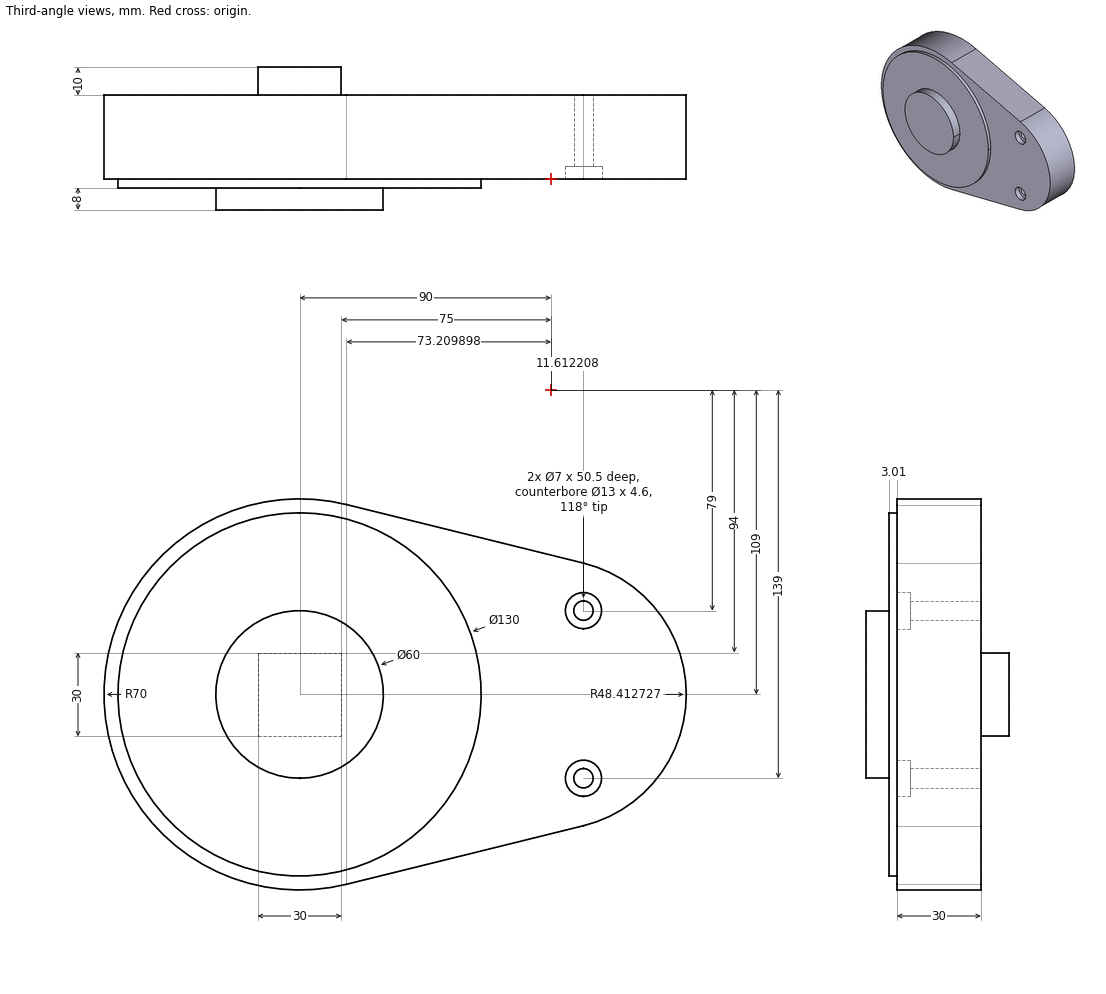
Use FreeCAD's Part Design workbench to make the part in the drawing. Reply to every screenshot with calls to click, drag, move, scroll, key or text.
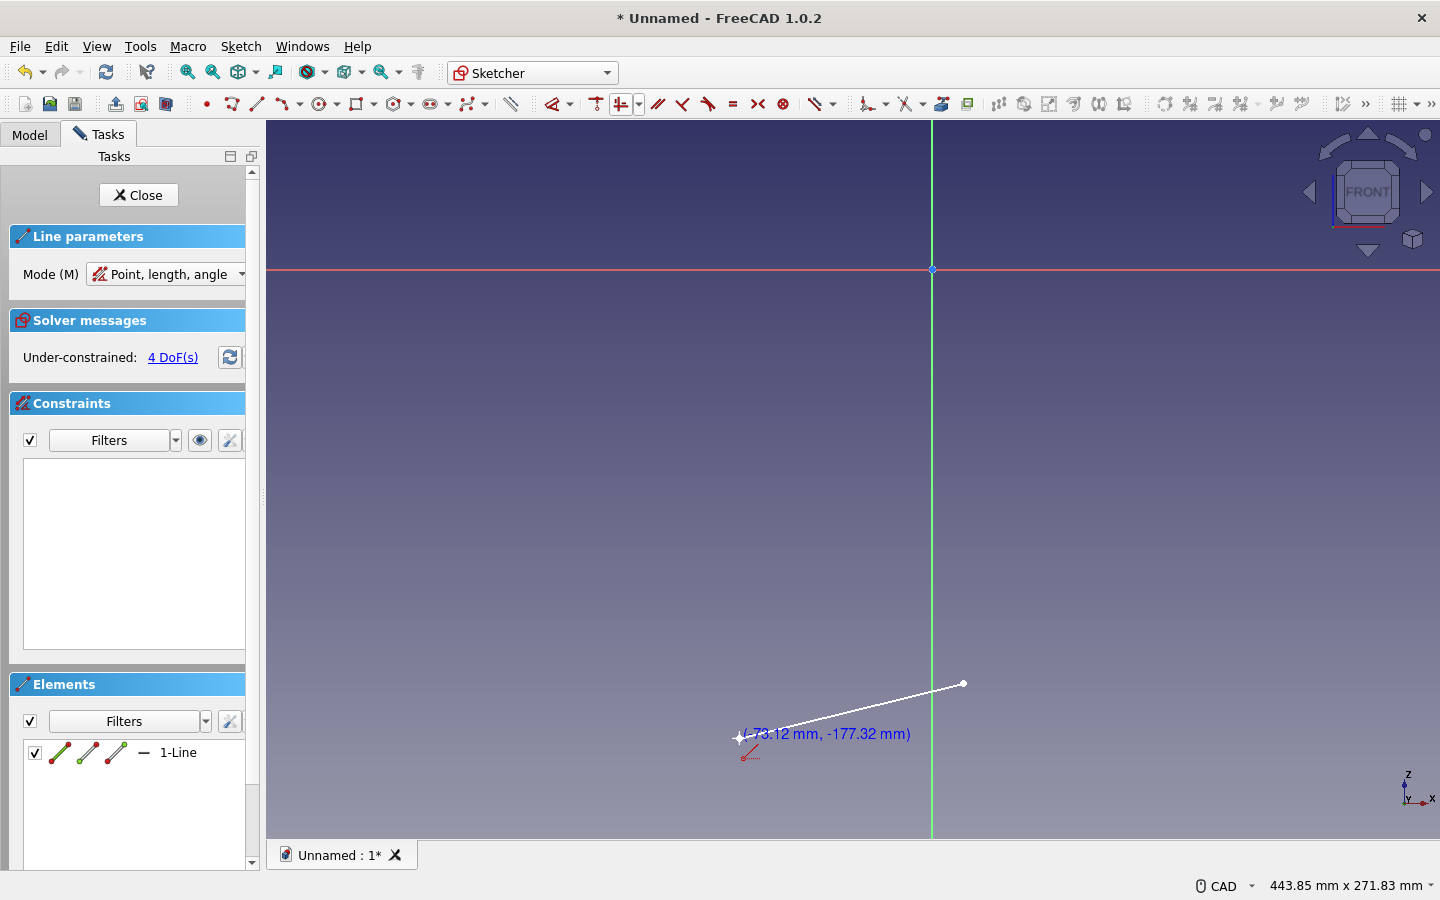
click(739, 379)
click(963, 434)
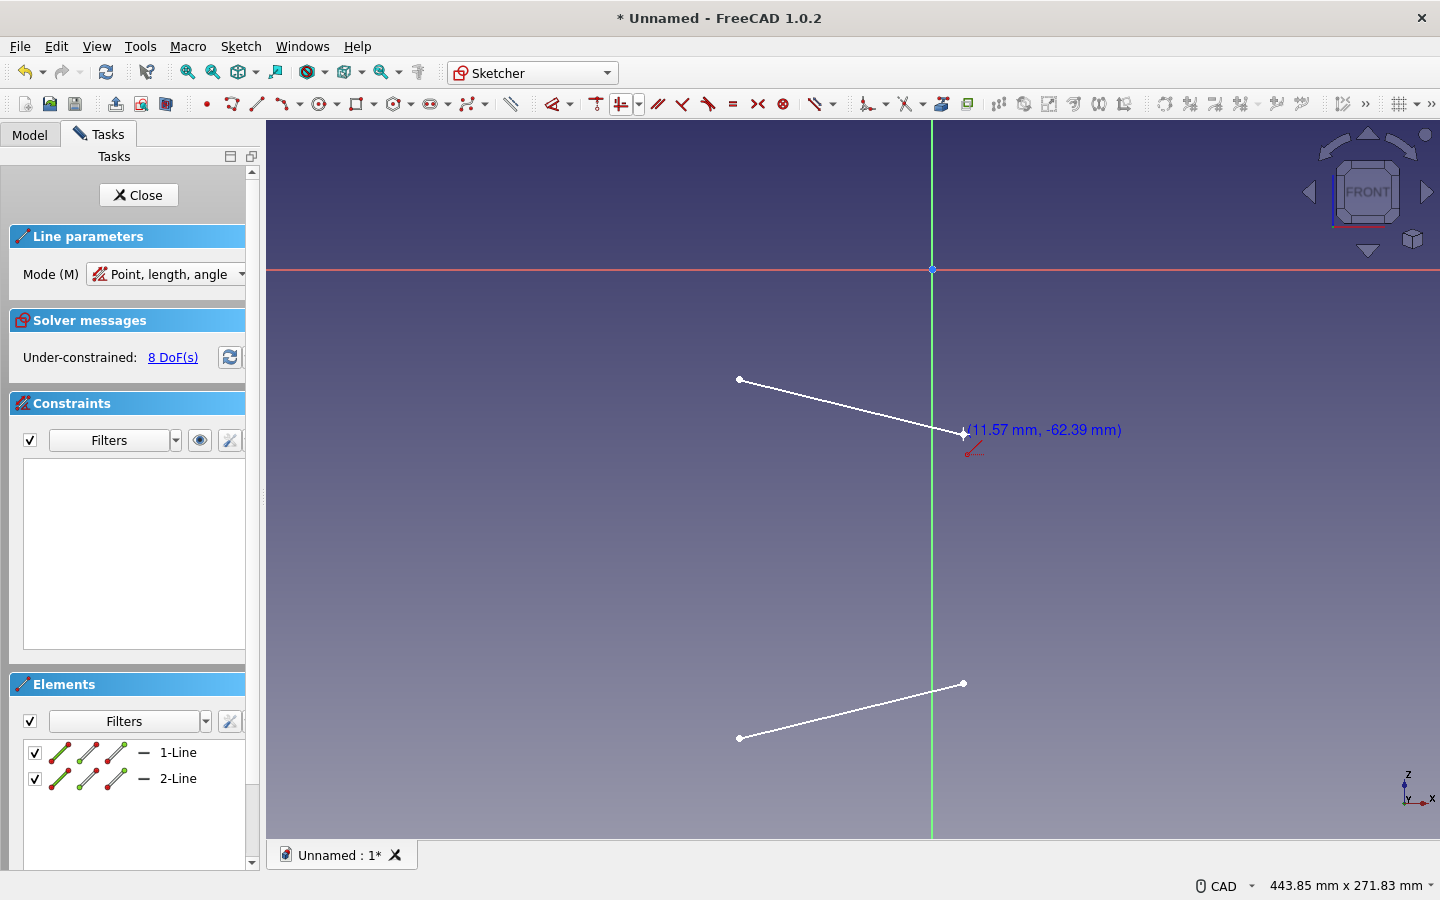
key(g)
key(3)
key(a)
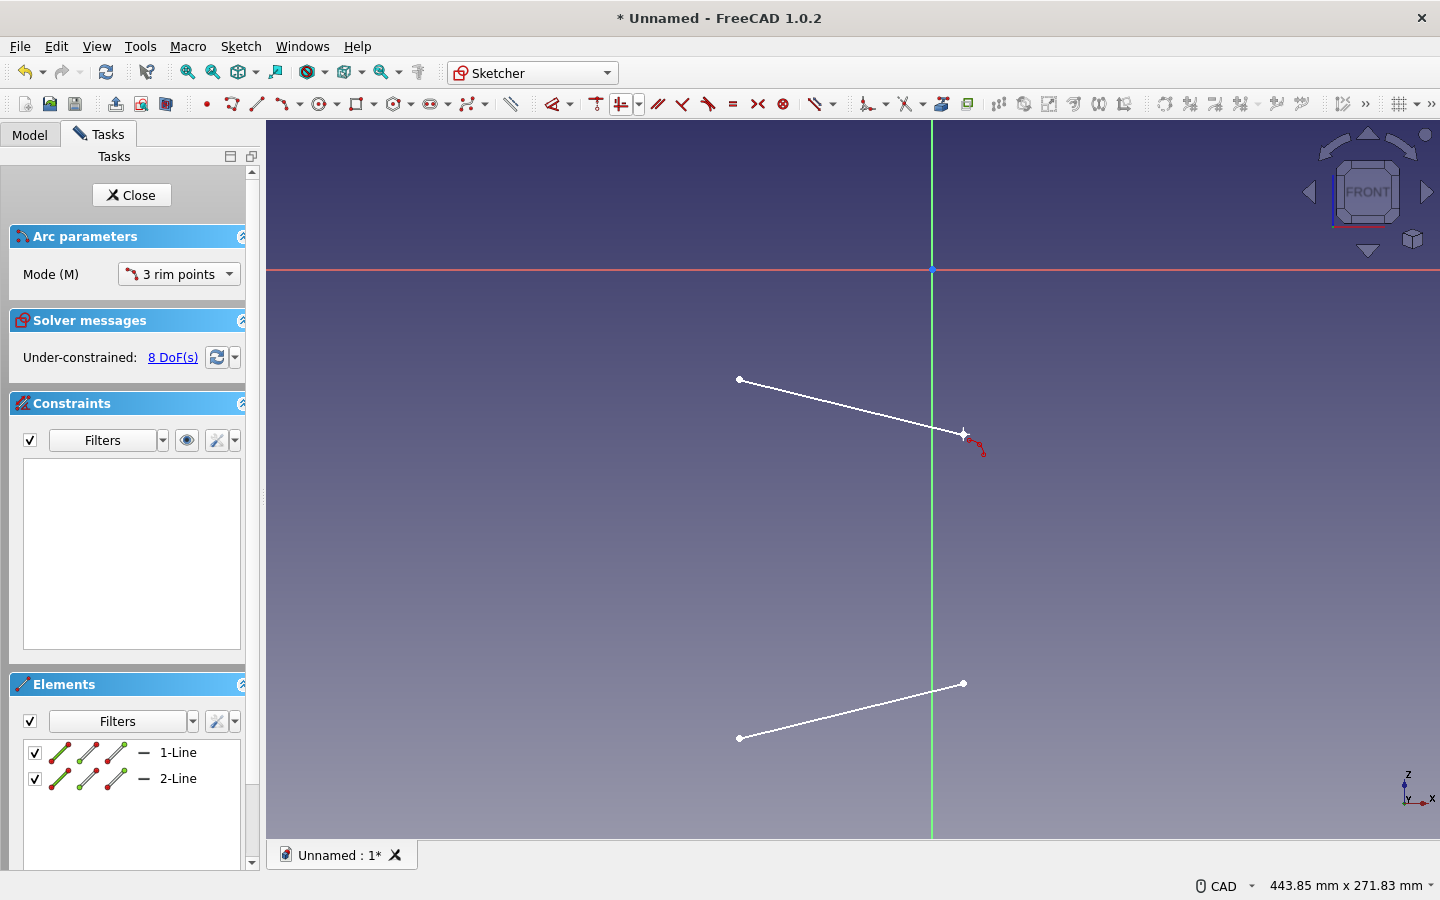
click(739, 739)
click(739, 380)
click(509, 558)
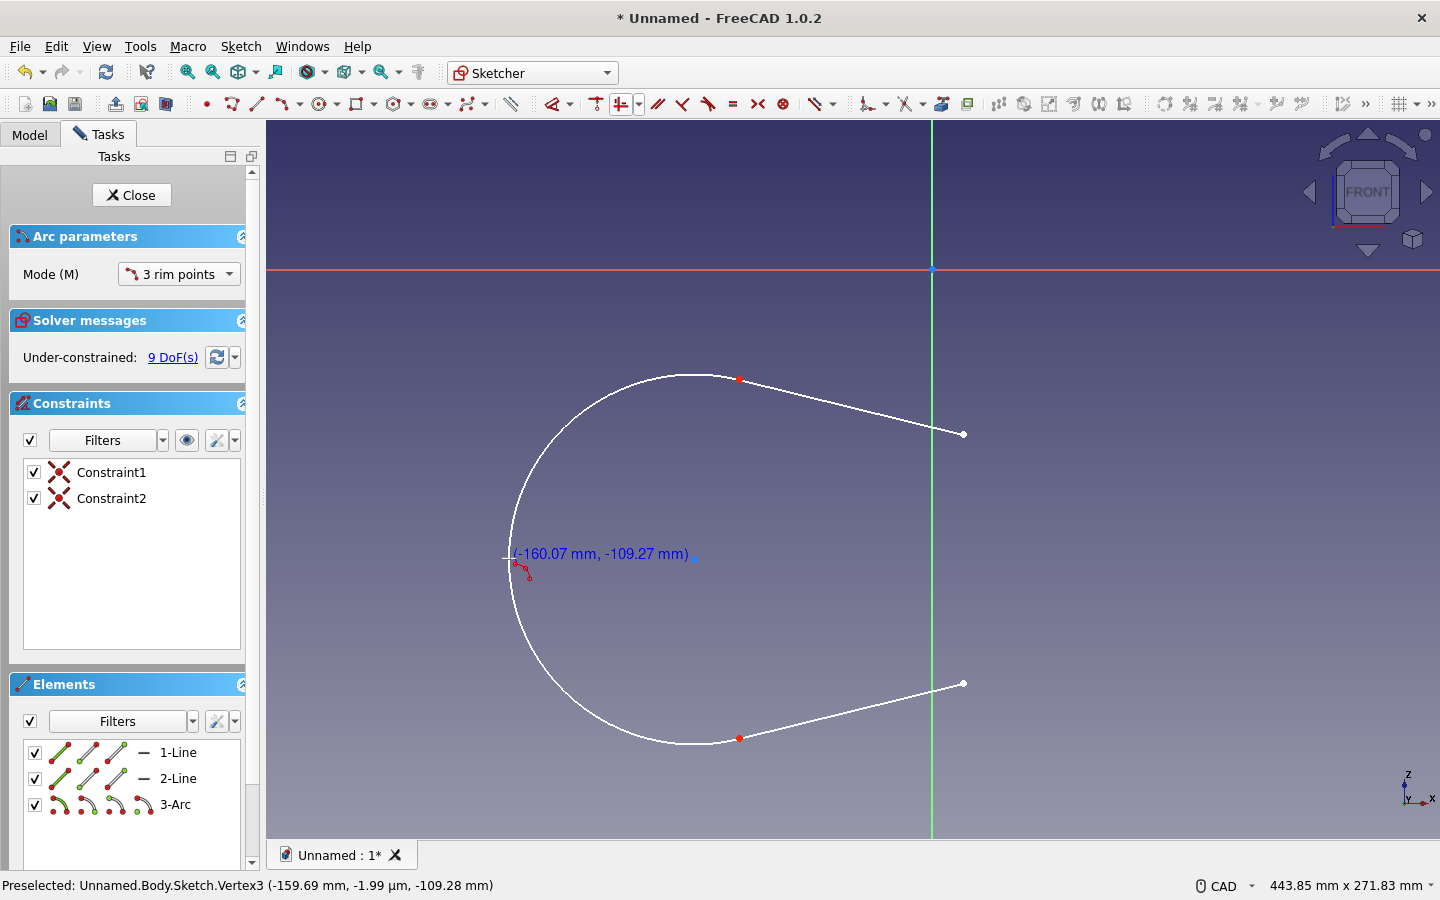
click(963, 435)
click(963, 684)
click(1060, 558)
key(Escape)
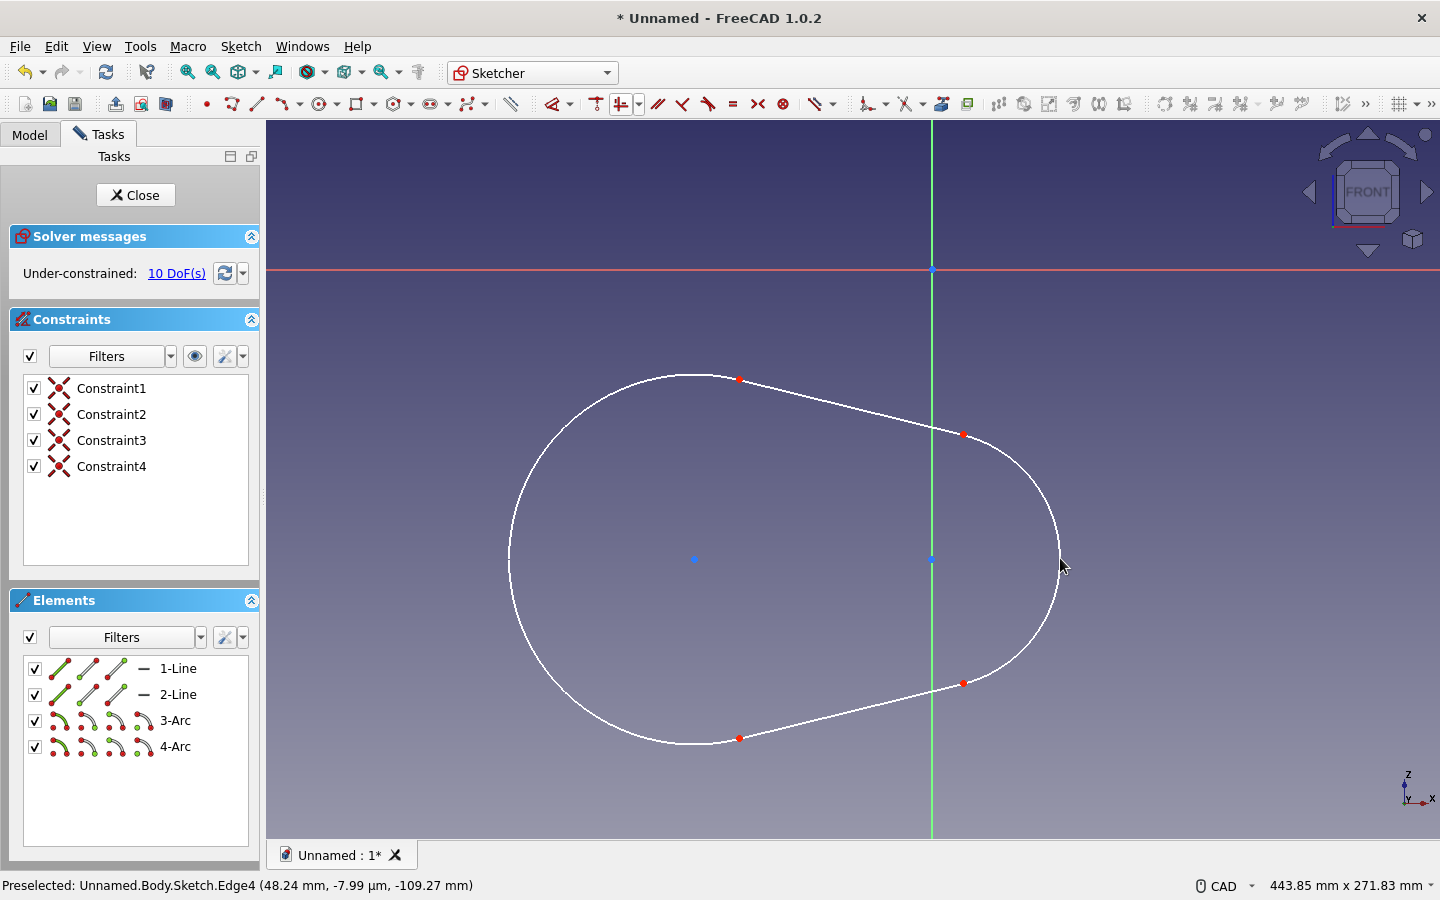
click(896, 701)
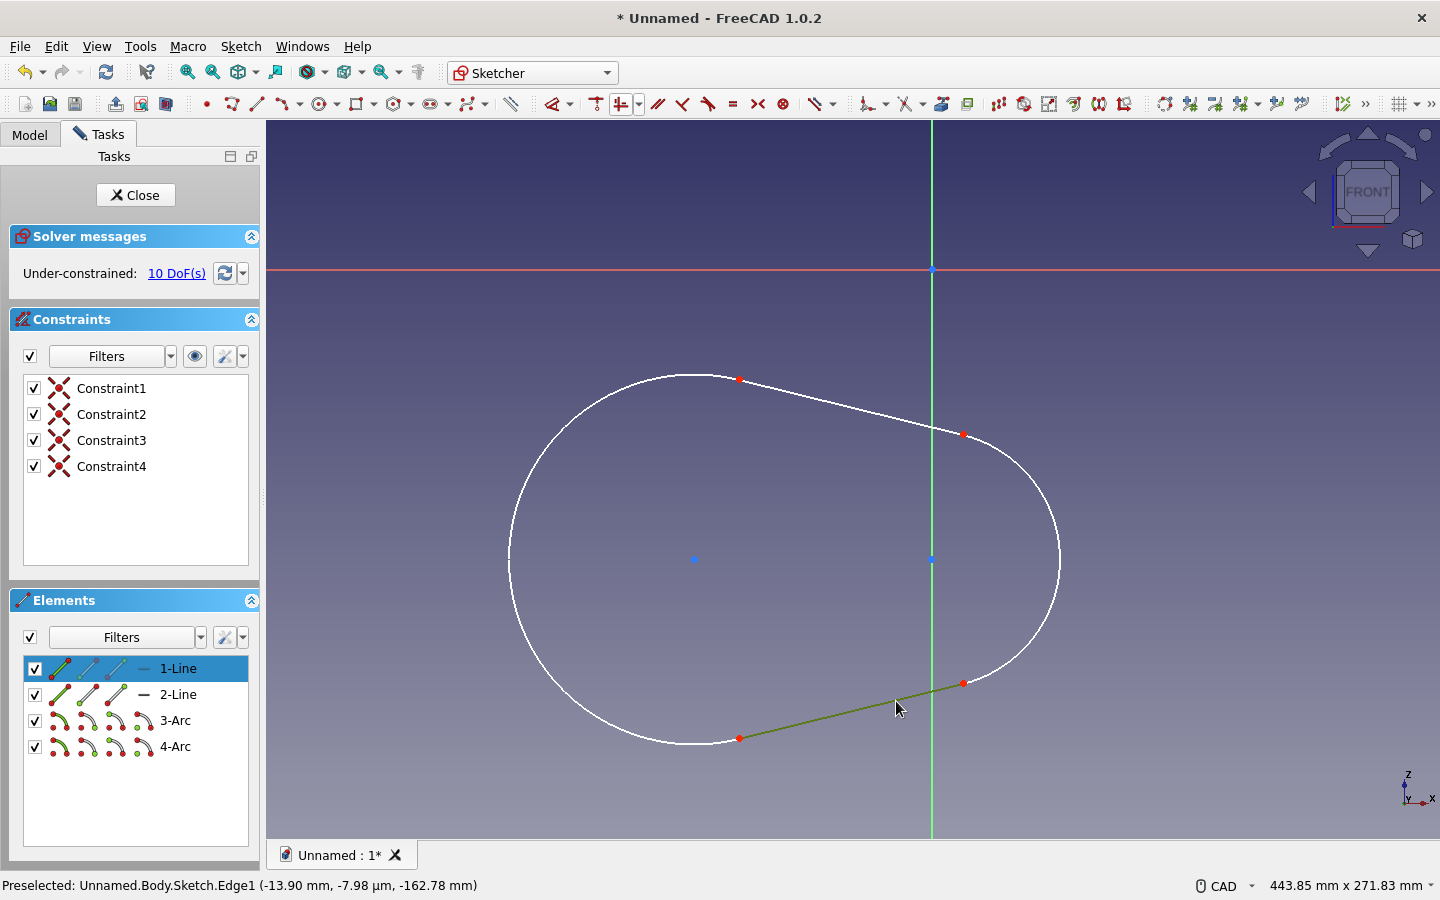
click(1042, 624)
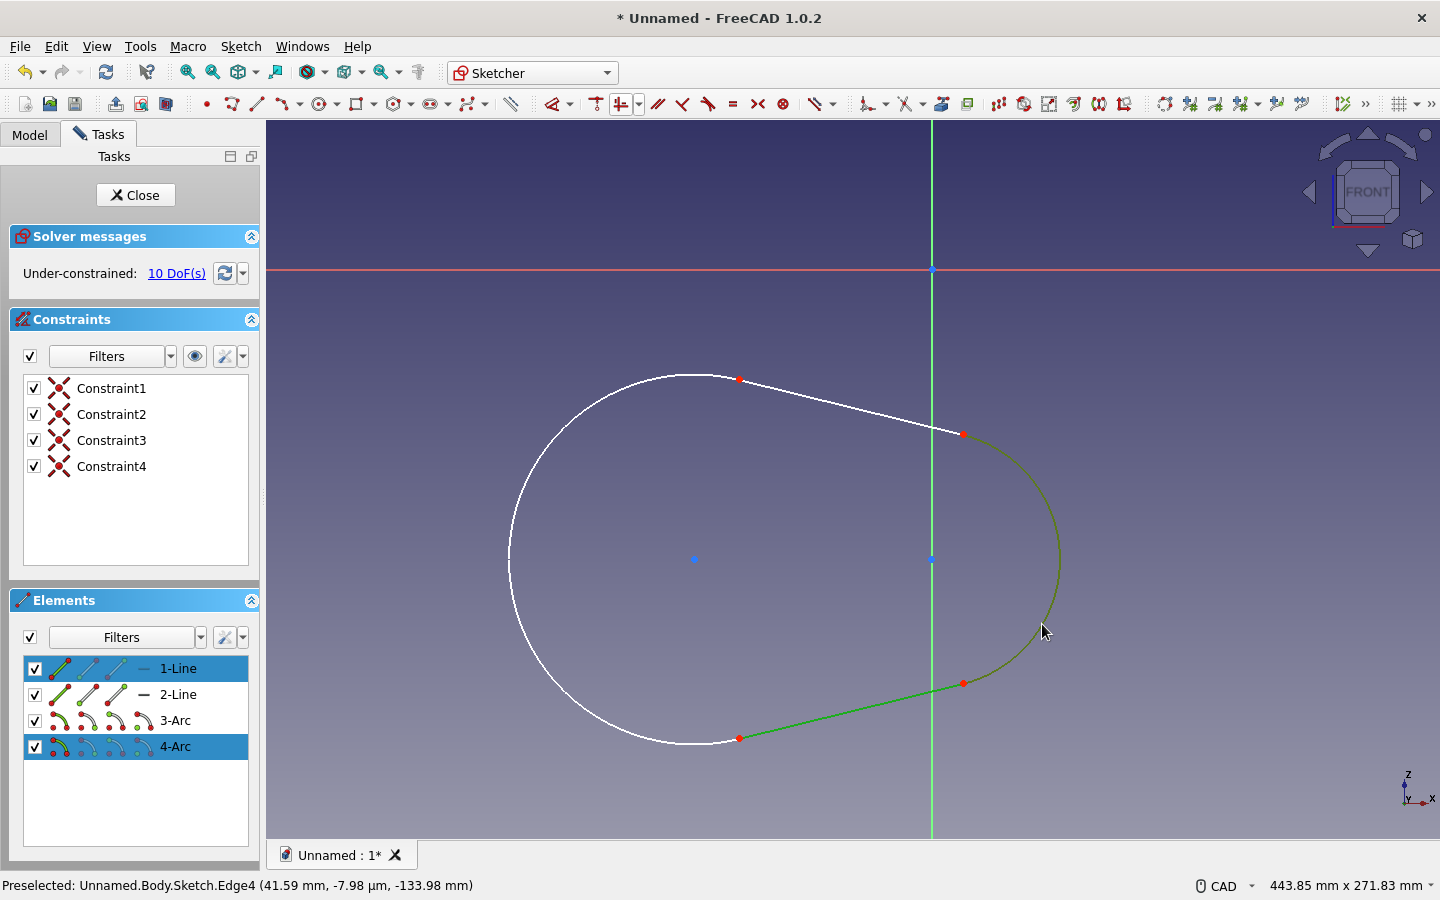
key(t)